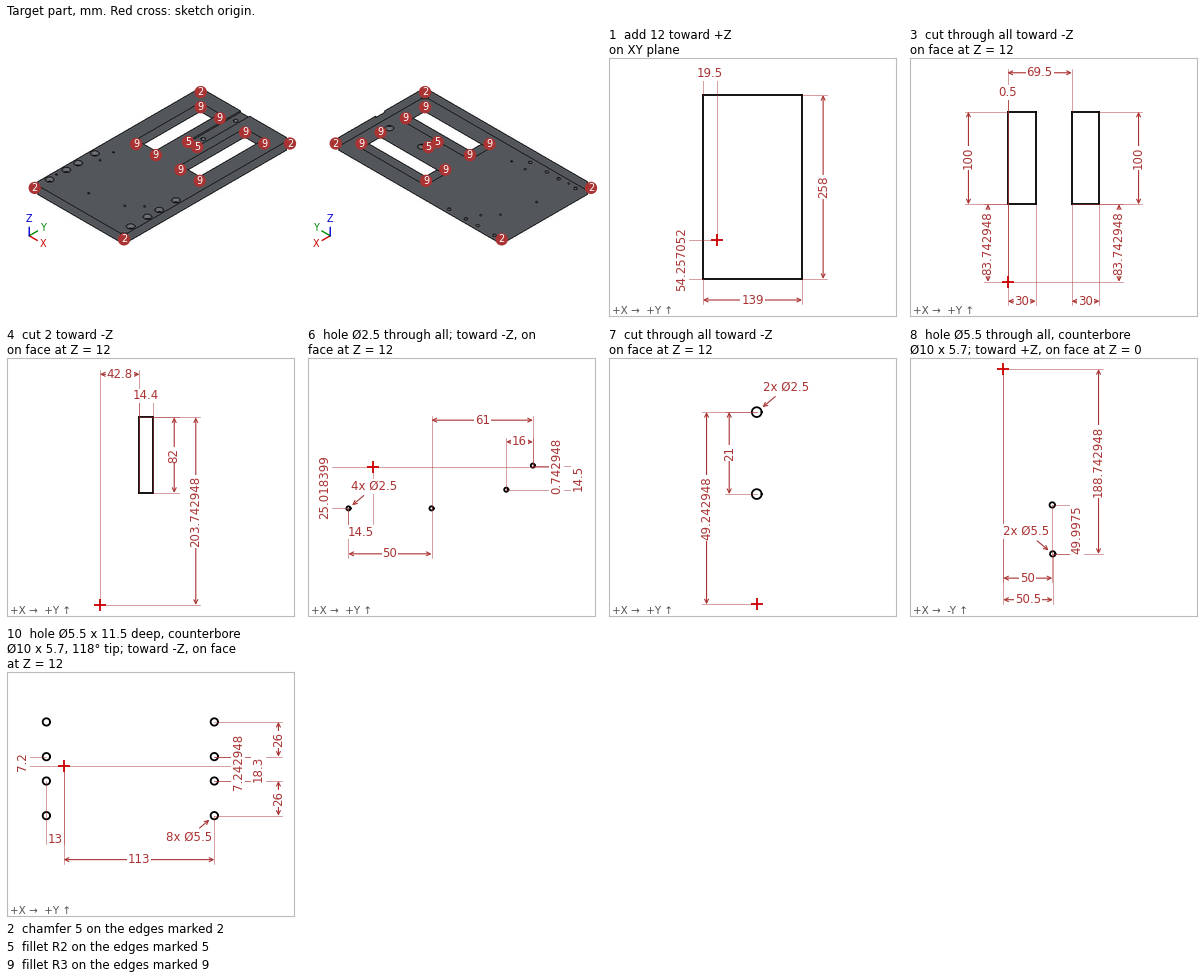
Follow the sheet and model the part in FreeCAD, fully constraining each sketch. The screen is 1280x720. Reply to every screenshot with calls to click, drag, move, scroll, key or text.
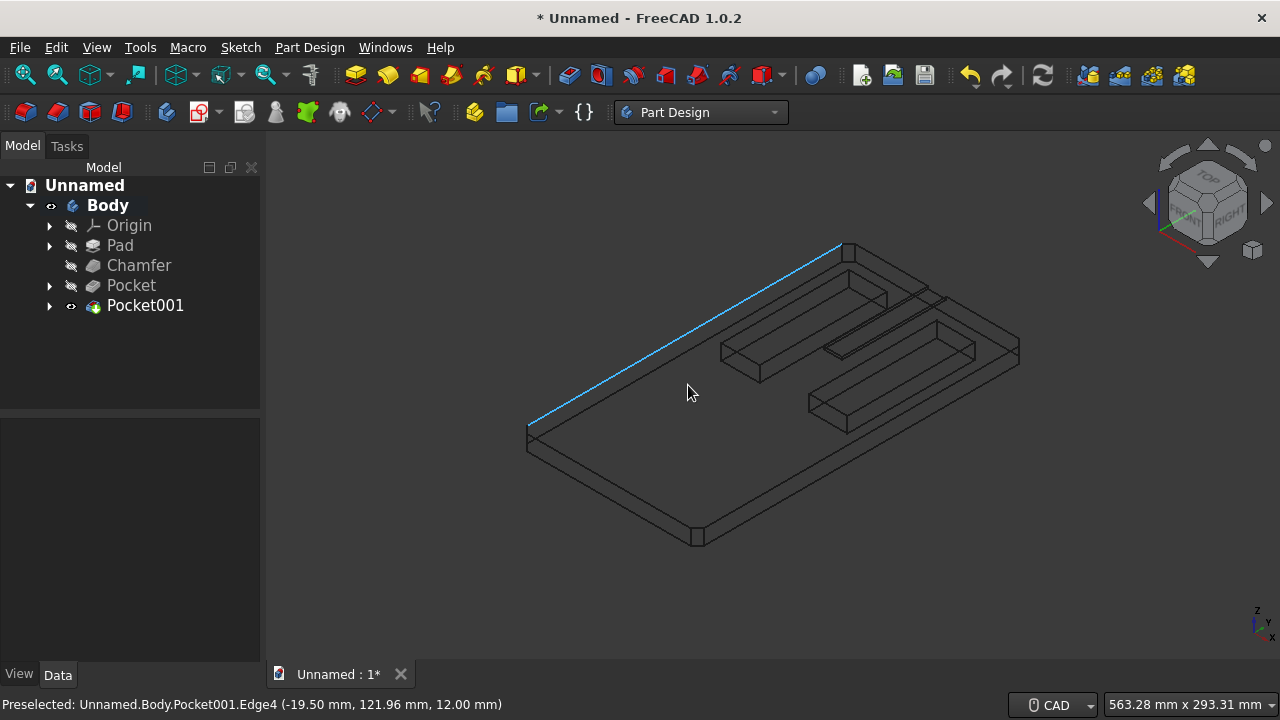
scroll(842, 357, up, 13)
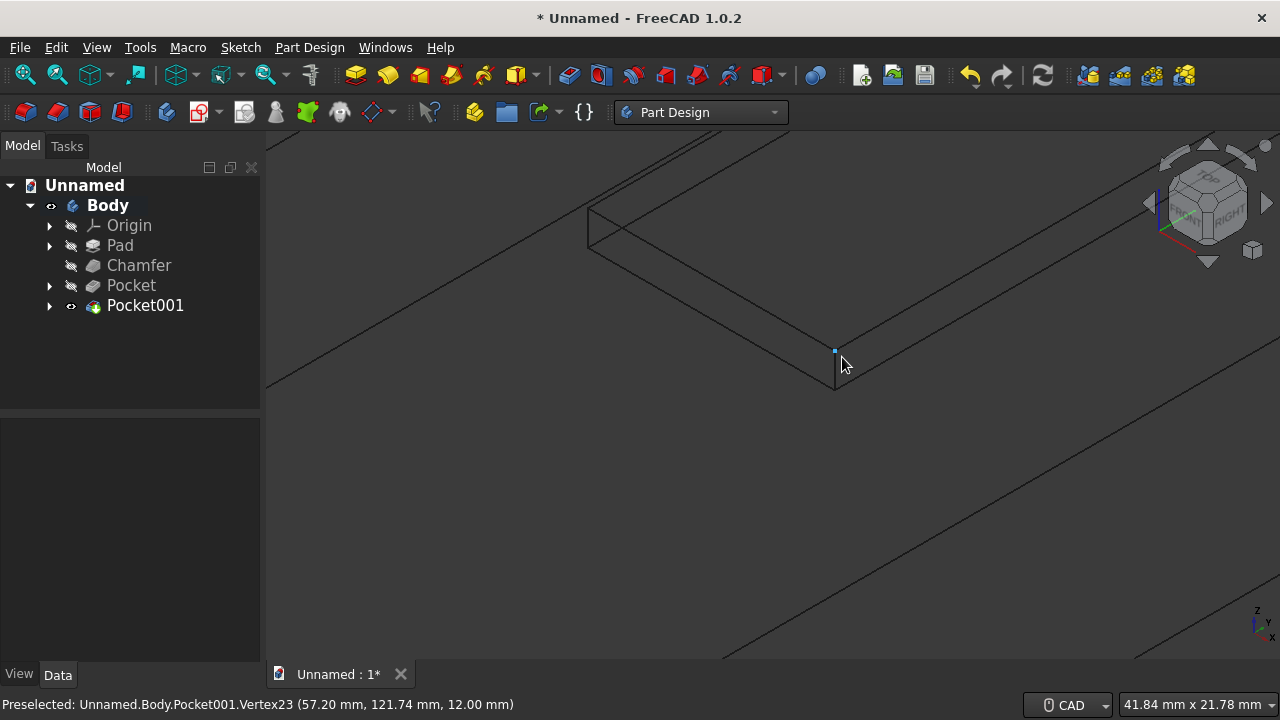
click(835, 370)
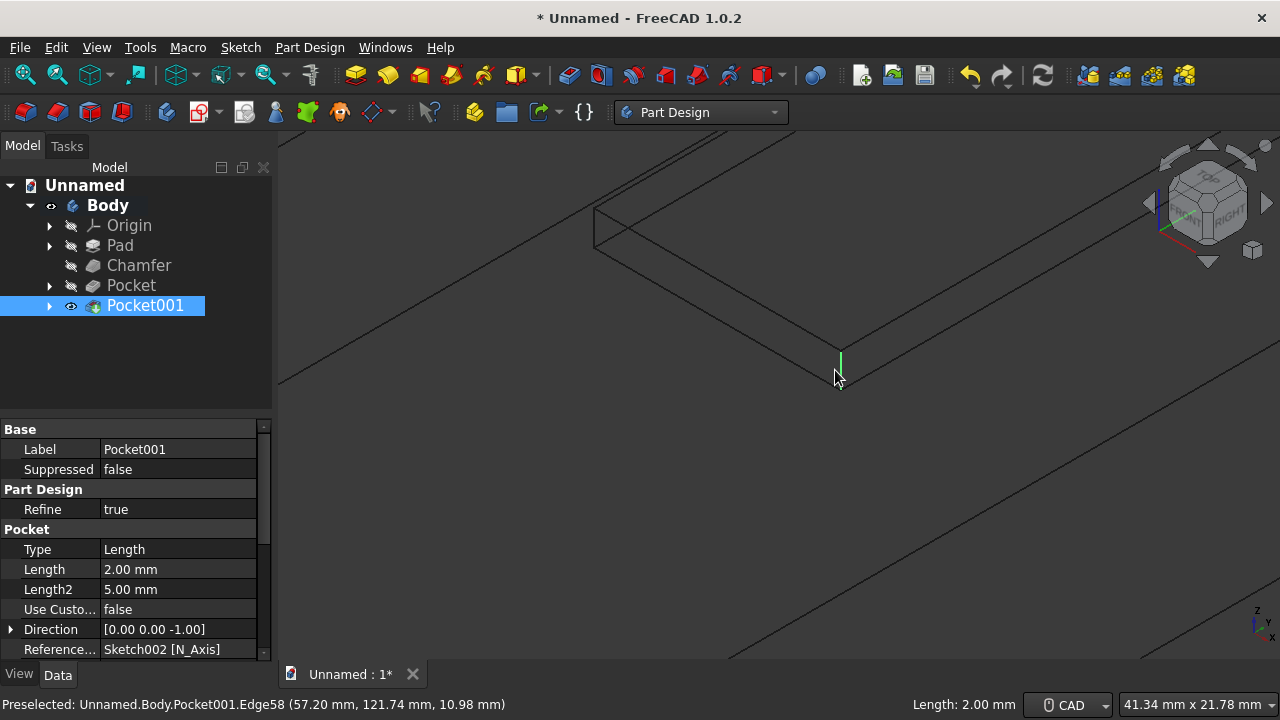
click(594, 227, ctrl)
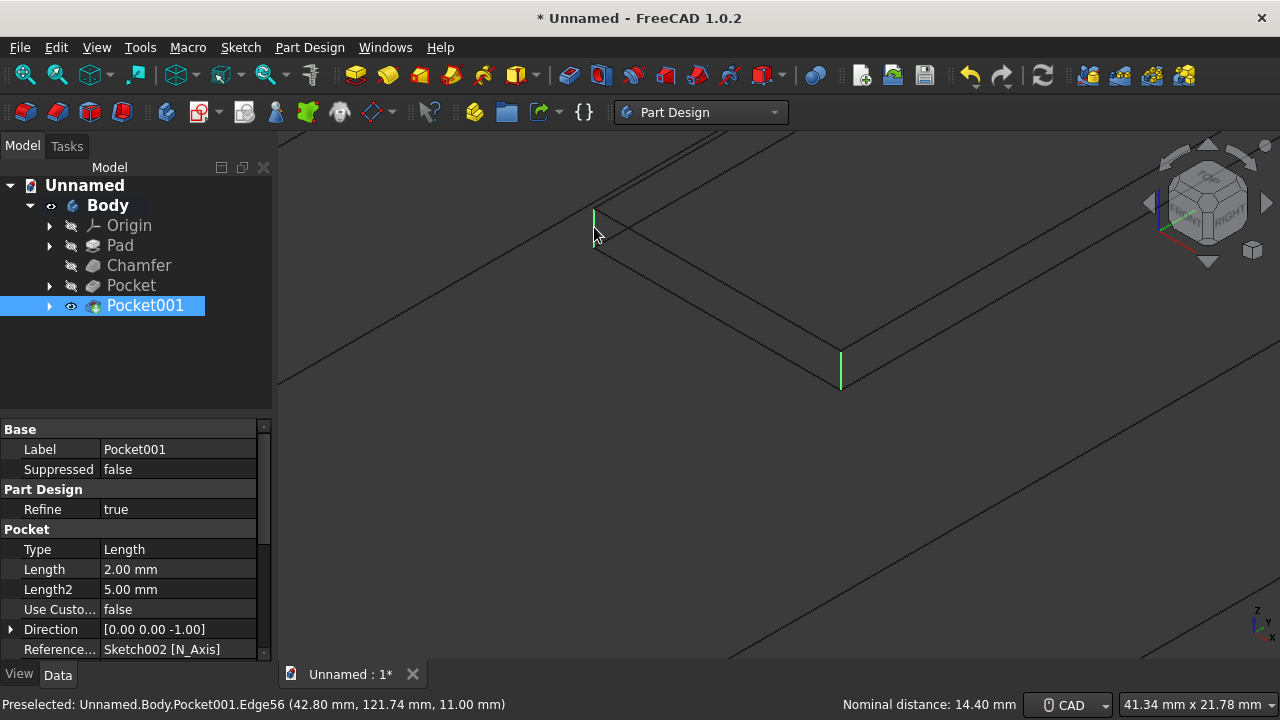
key(v)
key(1)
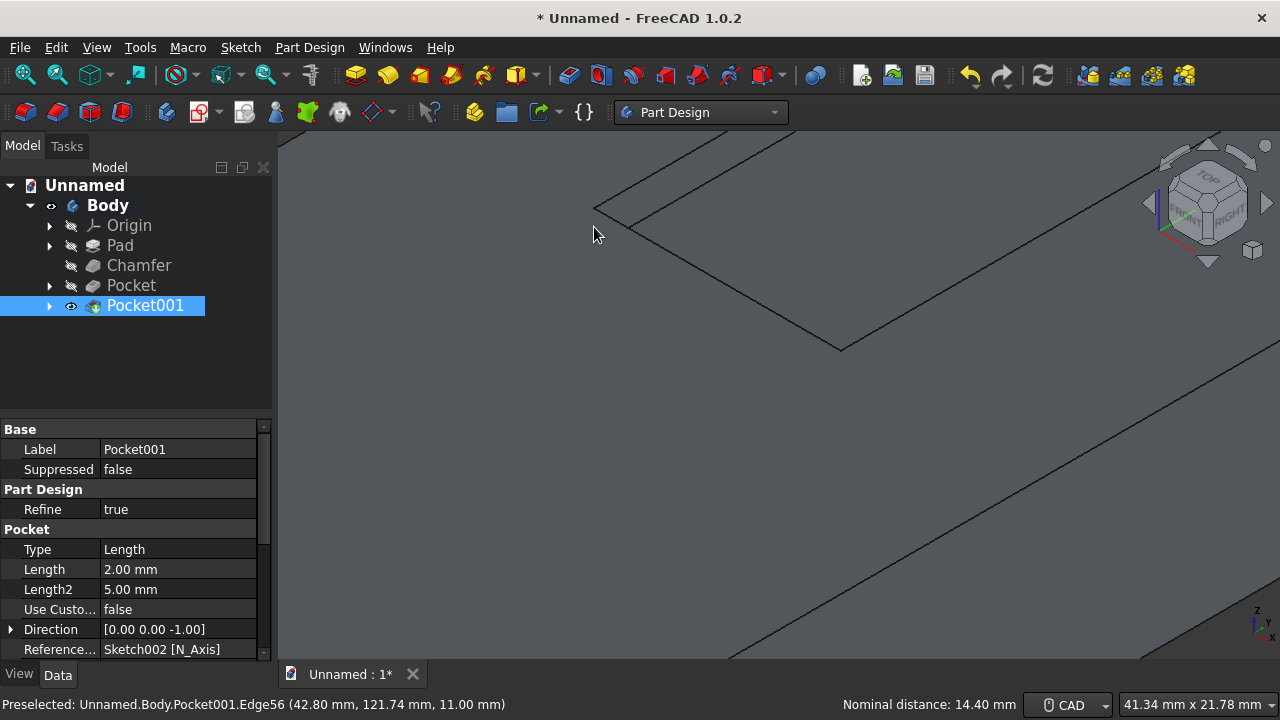
click(26, 112)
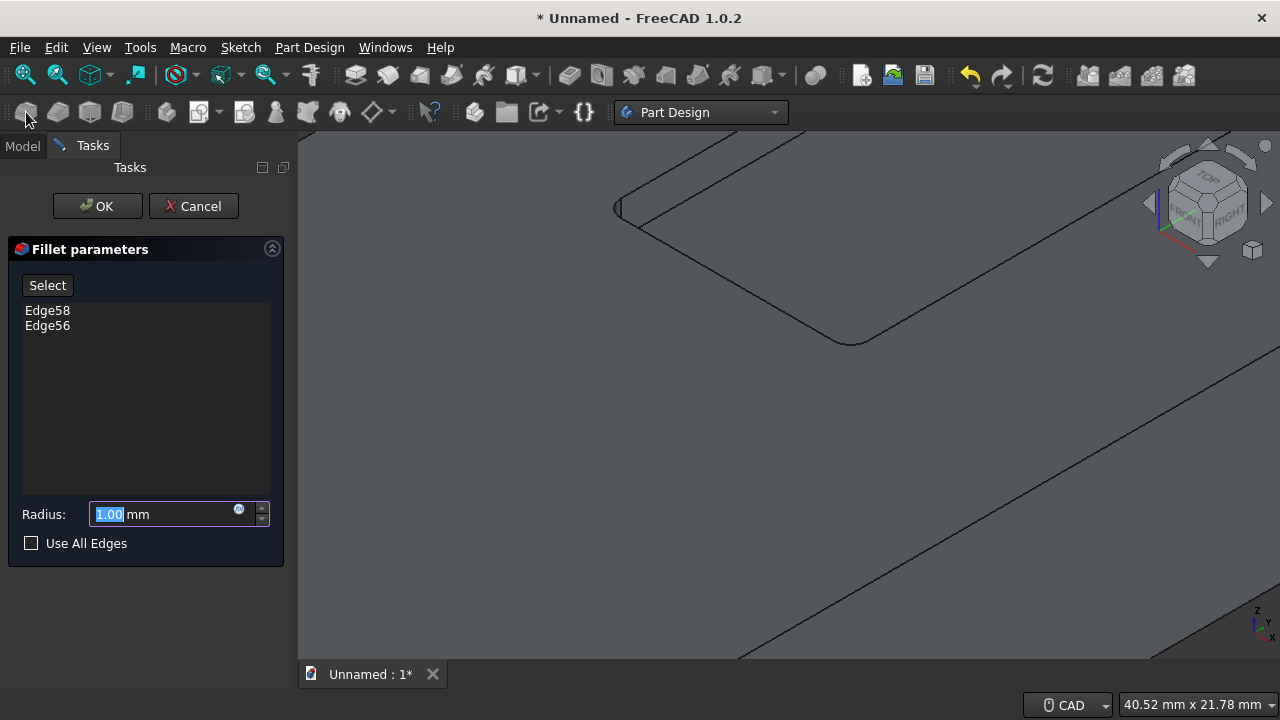
text(2)
key(Tab)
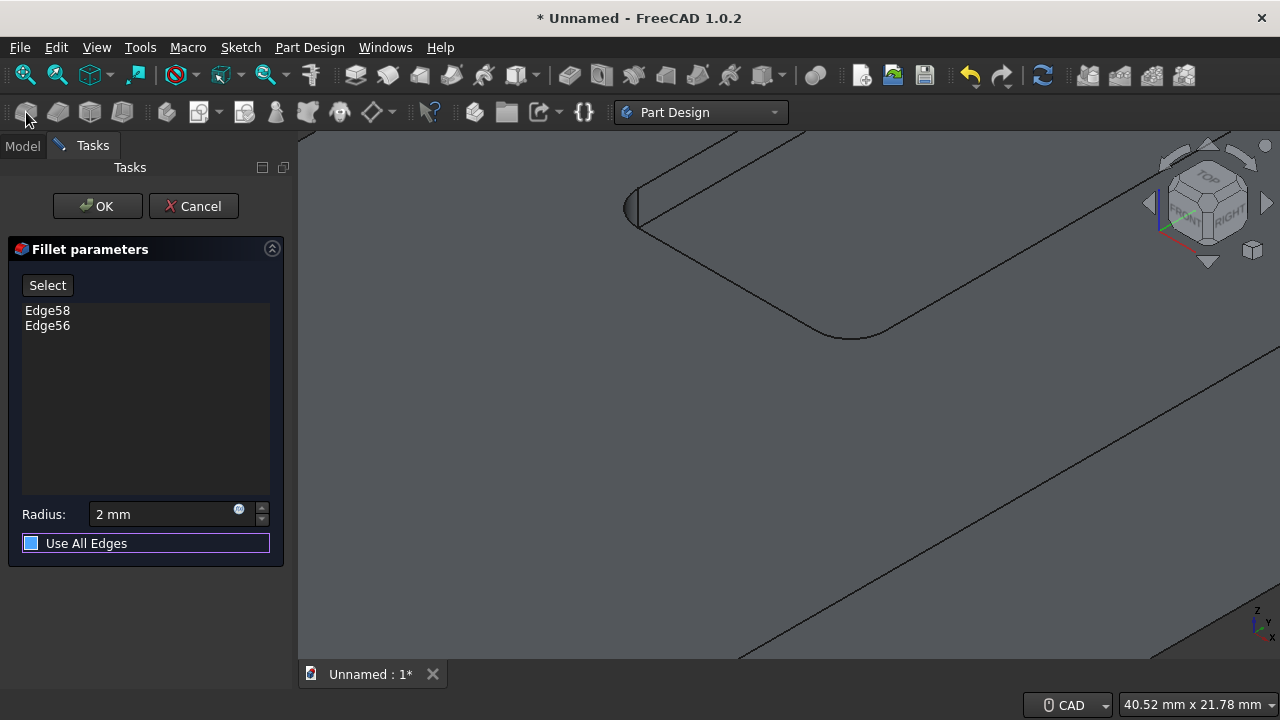
click(98, 206)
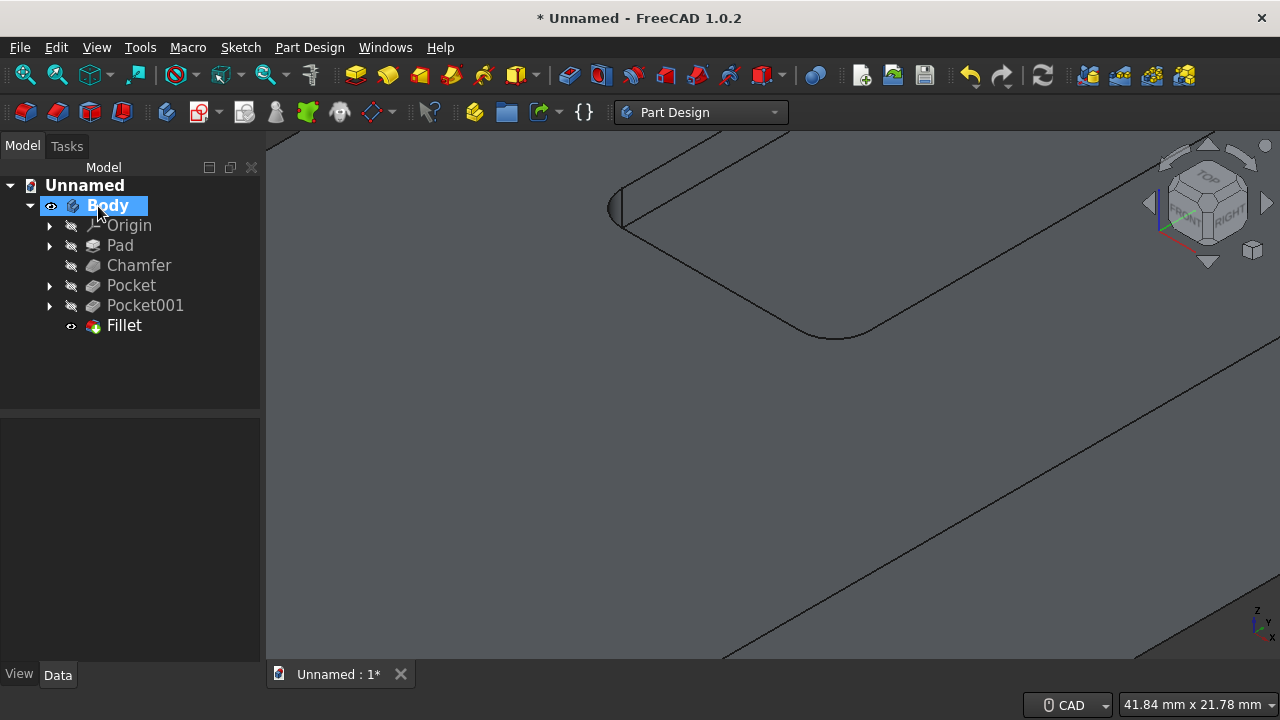
key(v)
key(f)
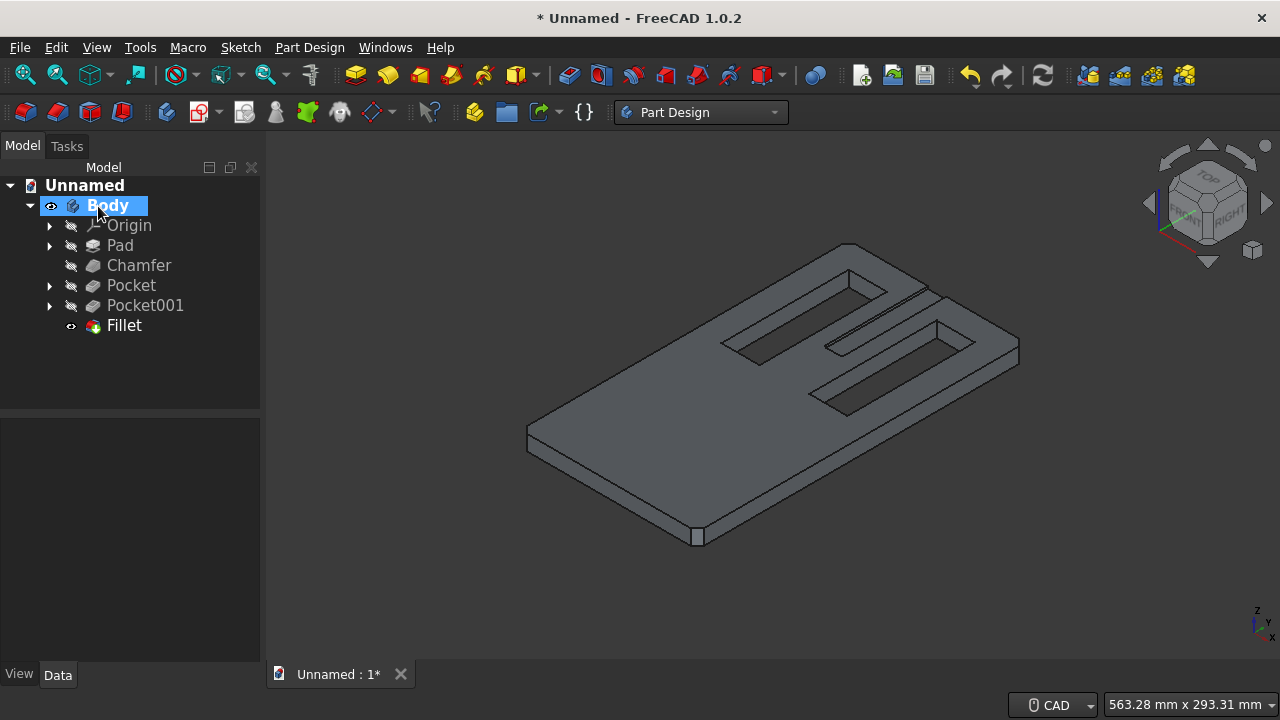
click(679, 439)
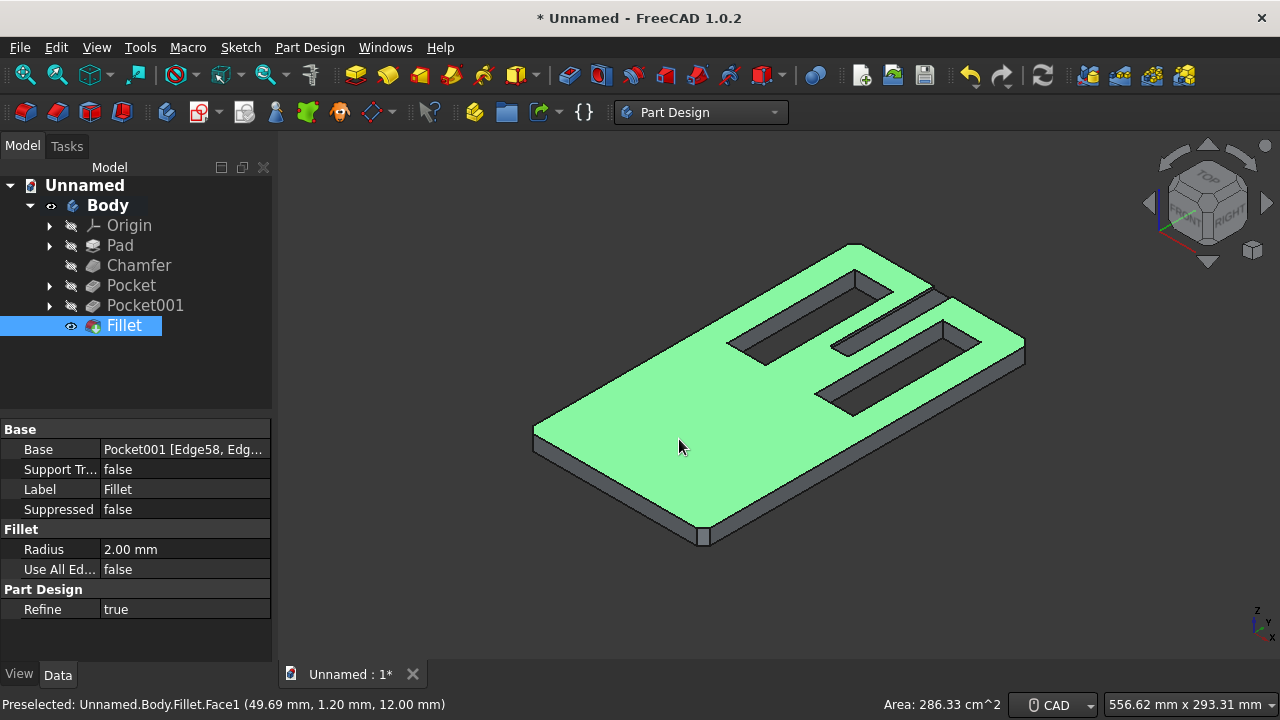
click(200, 112)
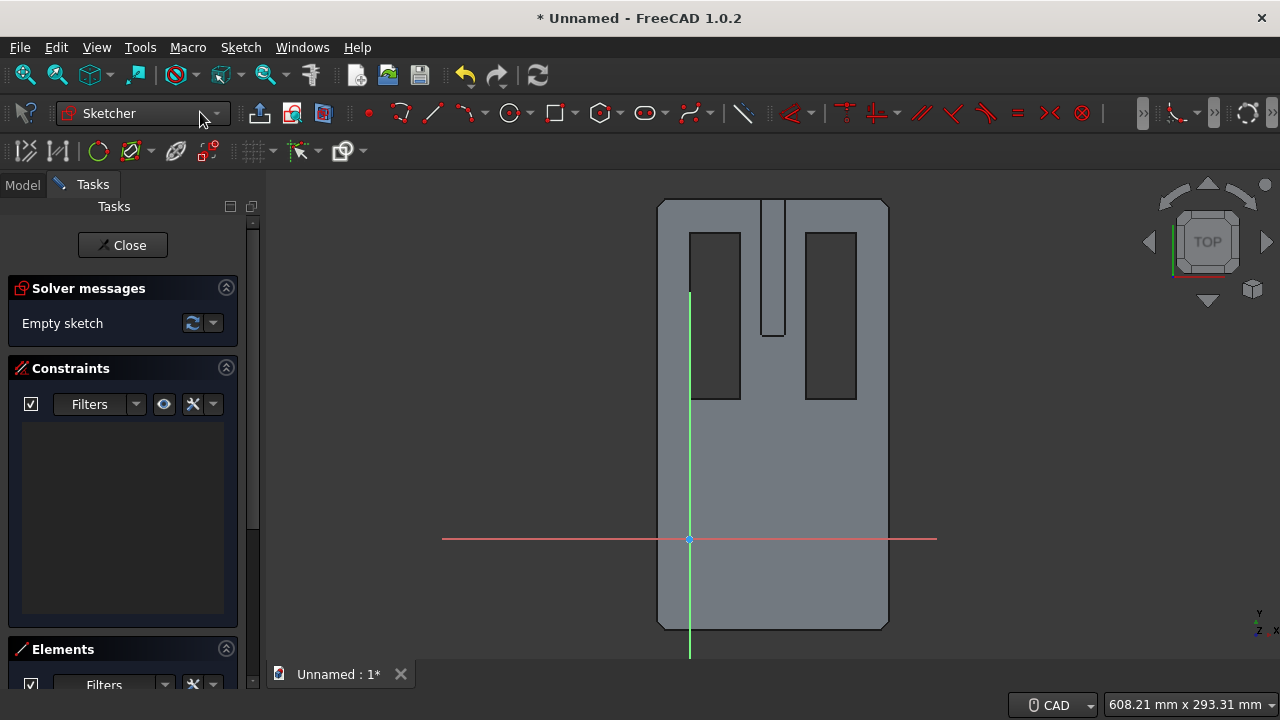
scroll(781, 622, up, 6)